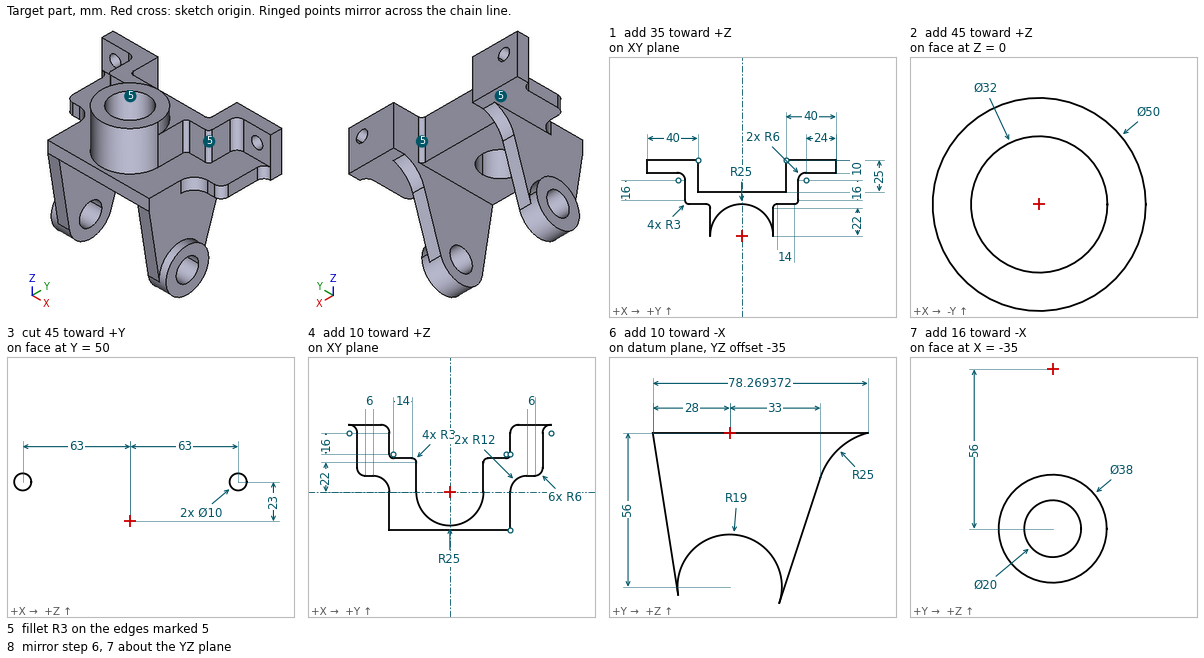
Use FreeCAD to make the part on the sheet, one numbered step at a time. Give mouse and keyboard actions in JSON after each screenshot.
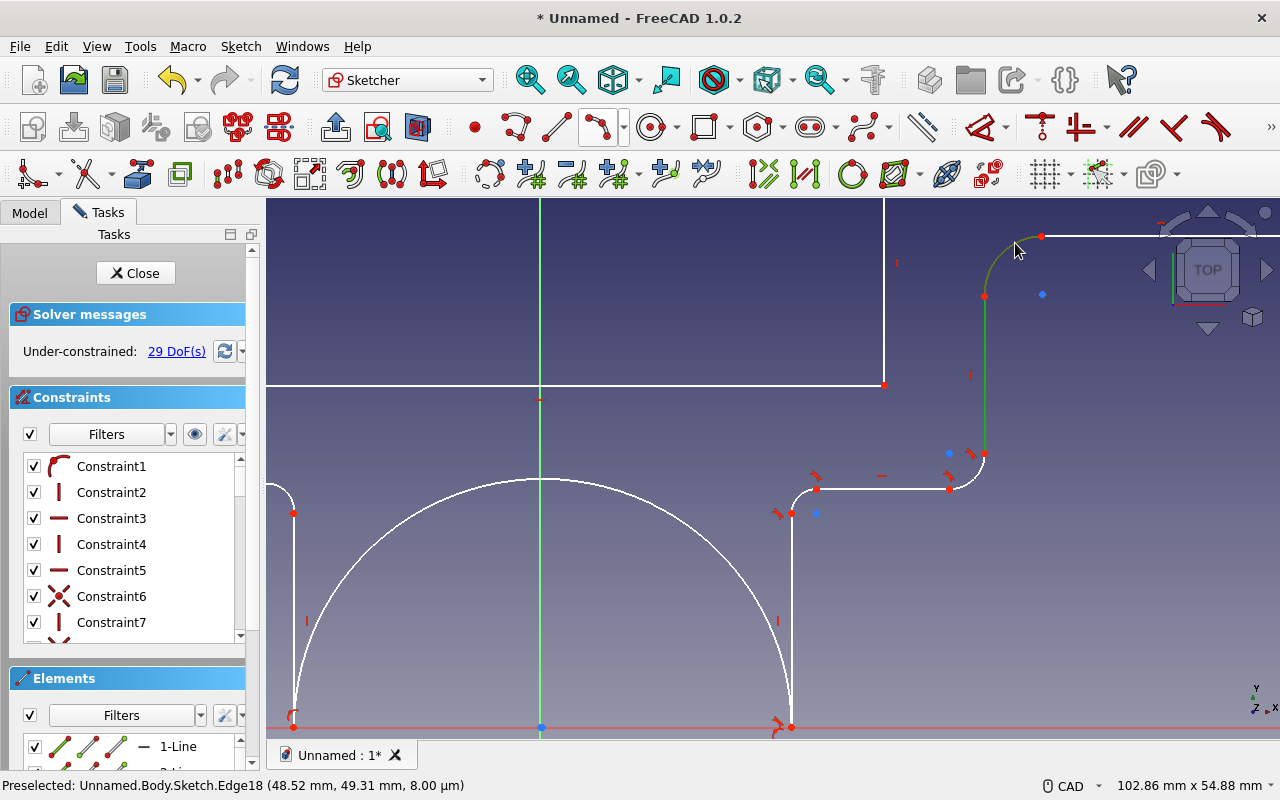
{"action": "left_click", "coordinate": [1216, 128]}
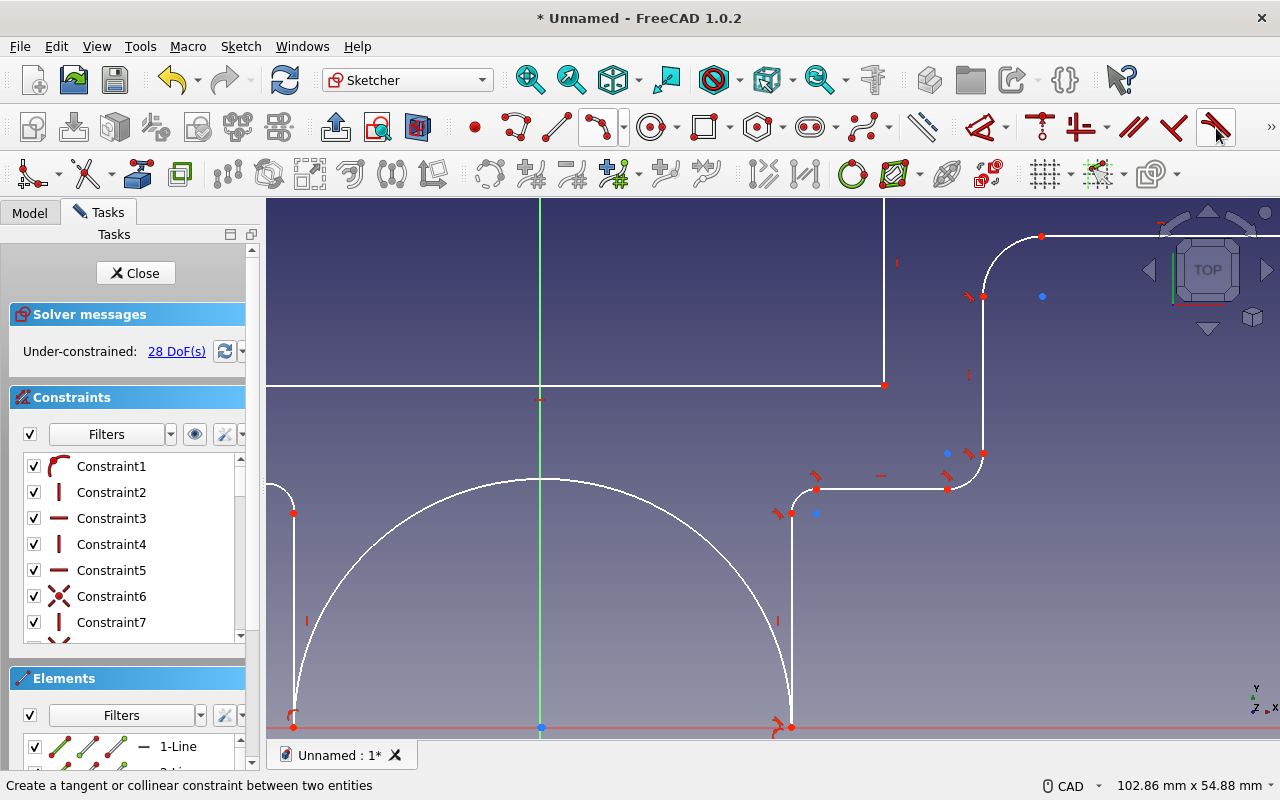
{"action": "left_click", "coordinate": [1114, 236]}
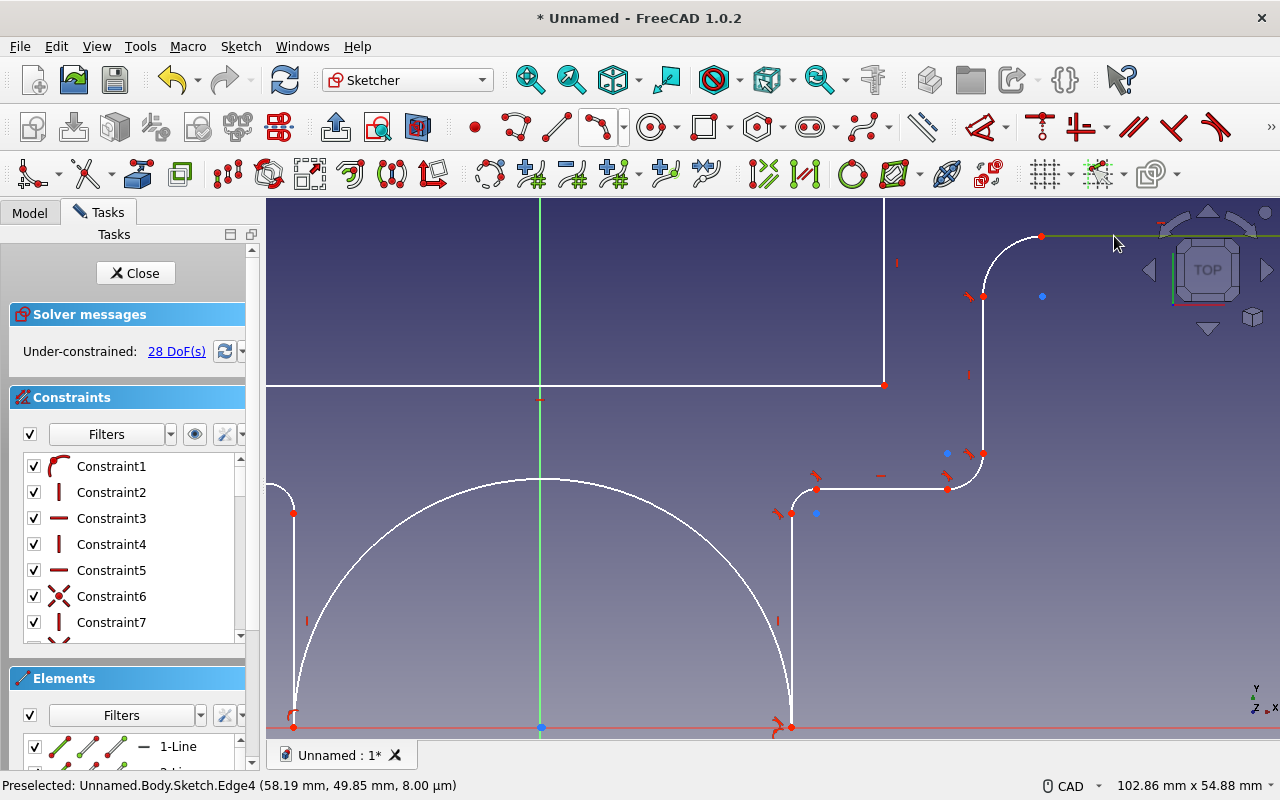
{"action": "left_click", "coordinate": [1015, 243]}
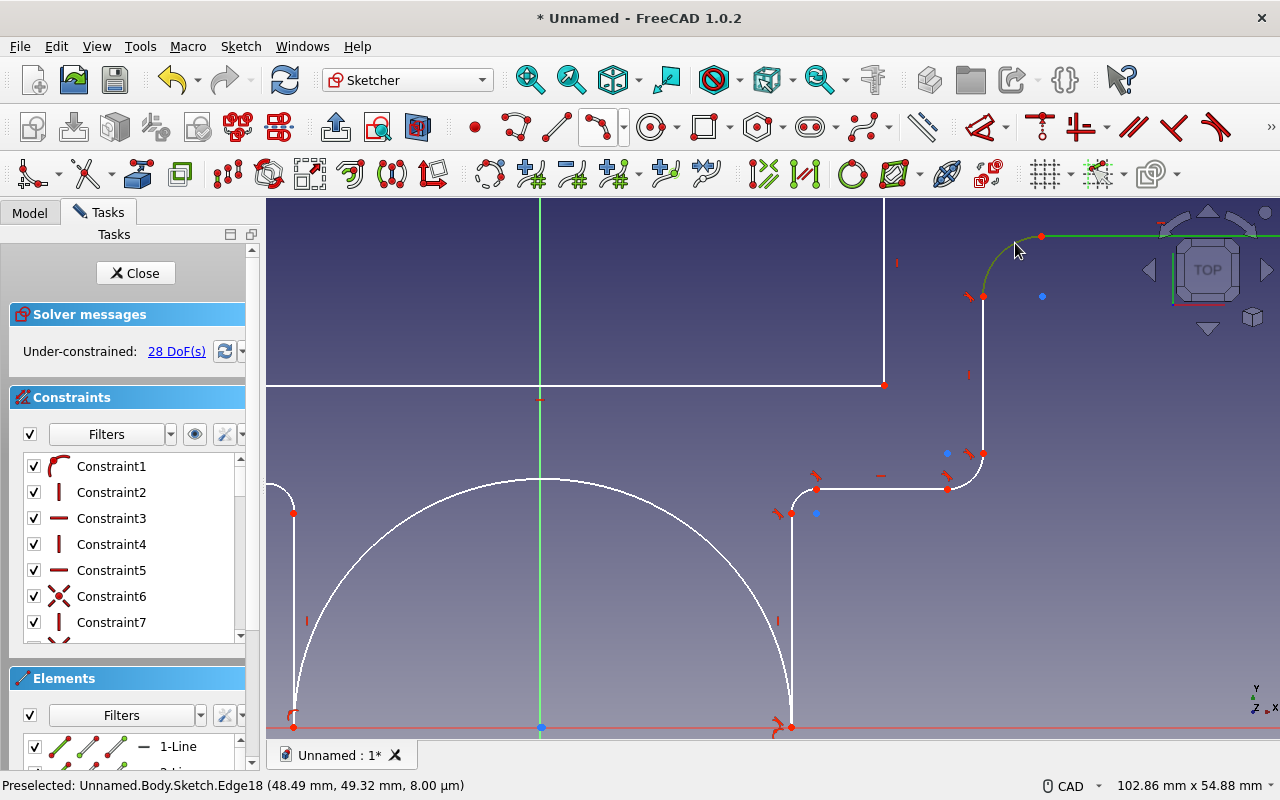
{"action": "left_click", "coordinate": [1216, 128]}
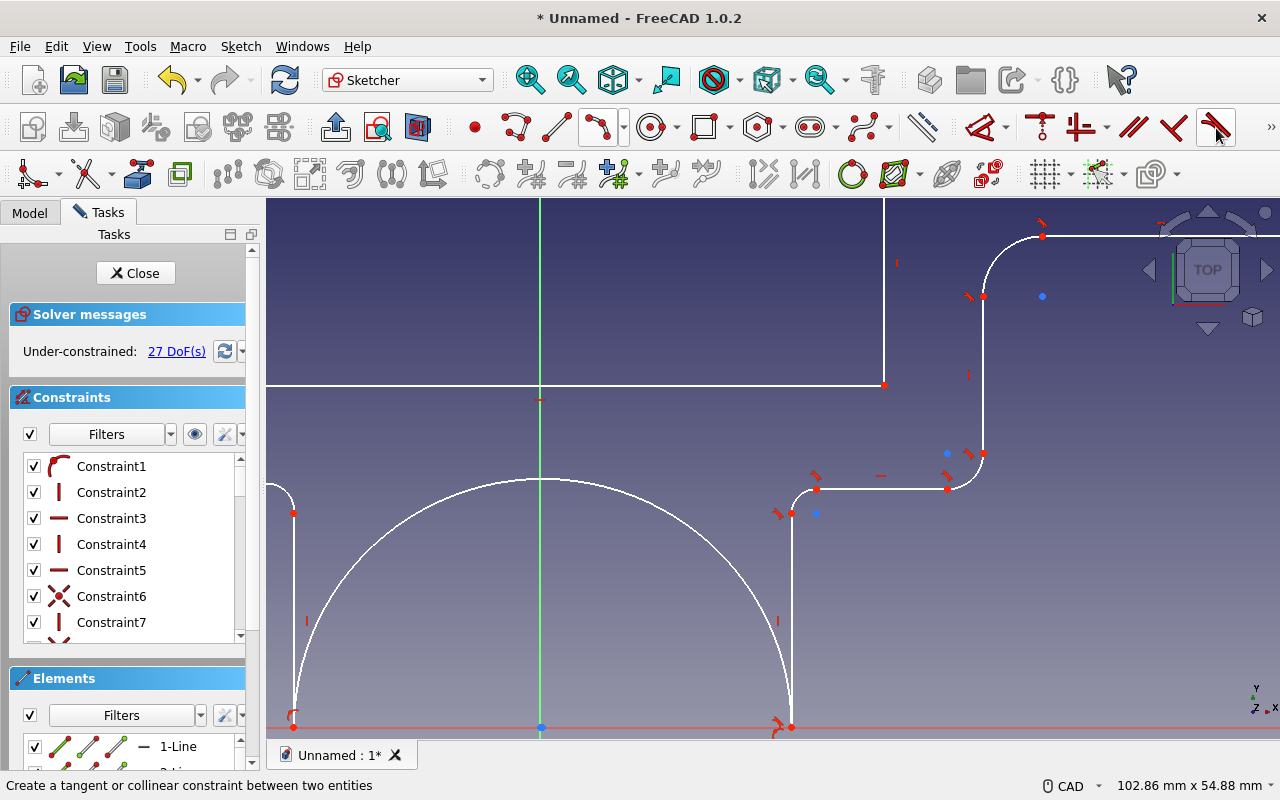
{"action": "scroll", "coordinate": [800, 490], "scroll_direction": "down", "scroll_amount": 5}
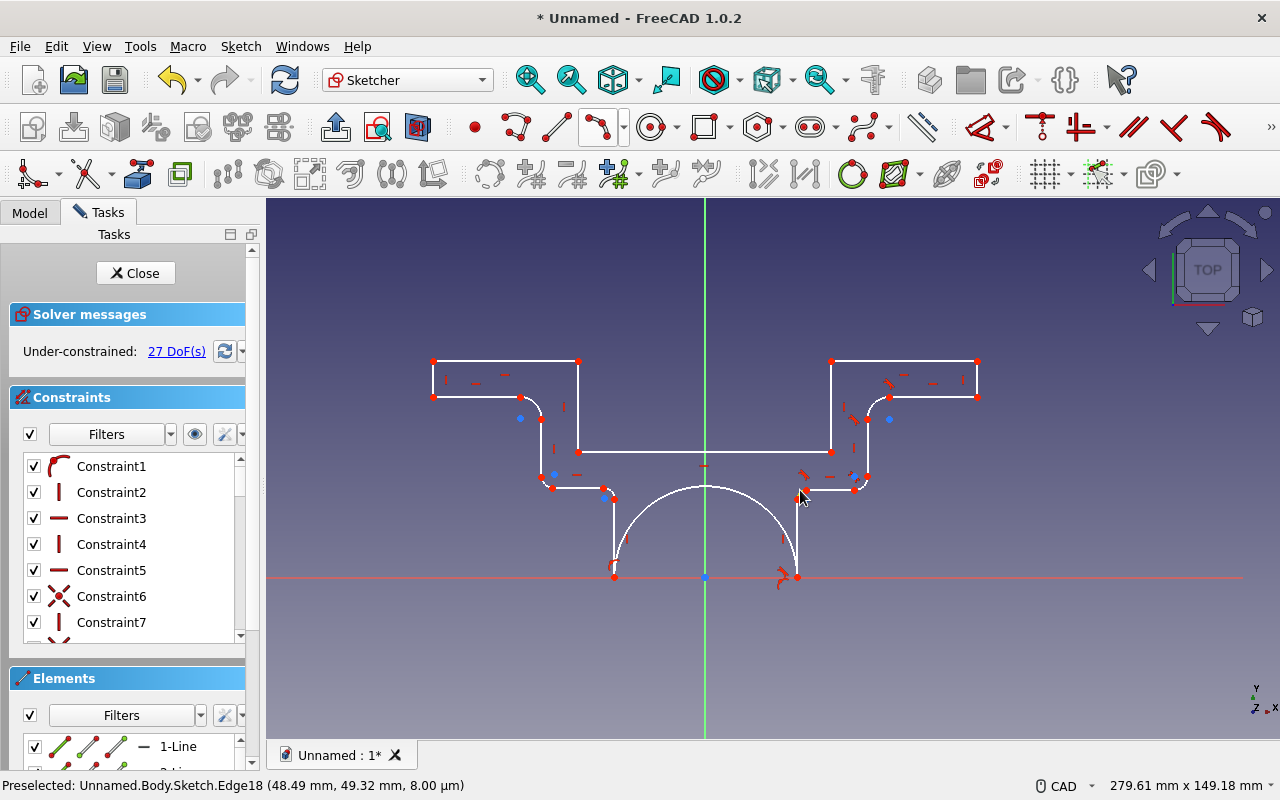
{"action": "left_click", "coordinate": [459, 397]}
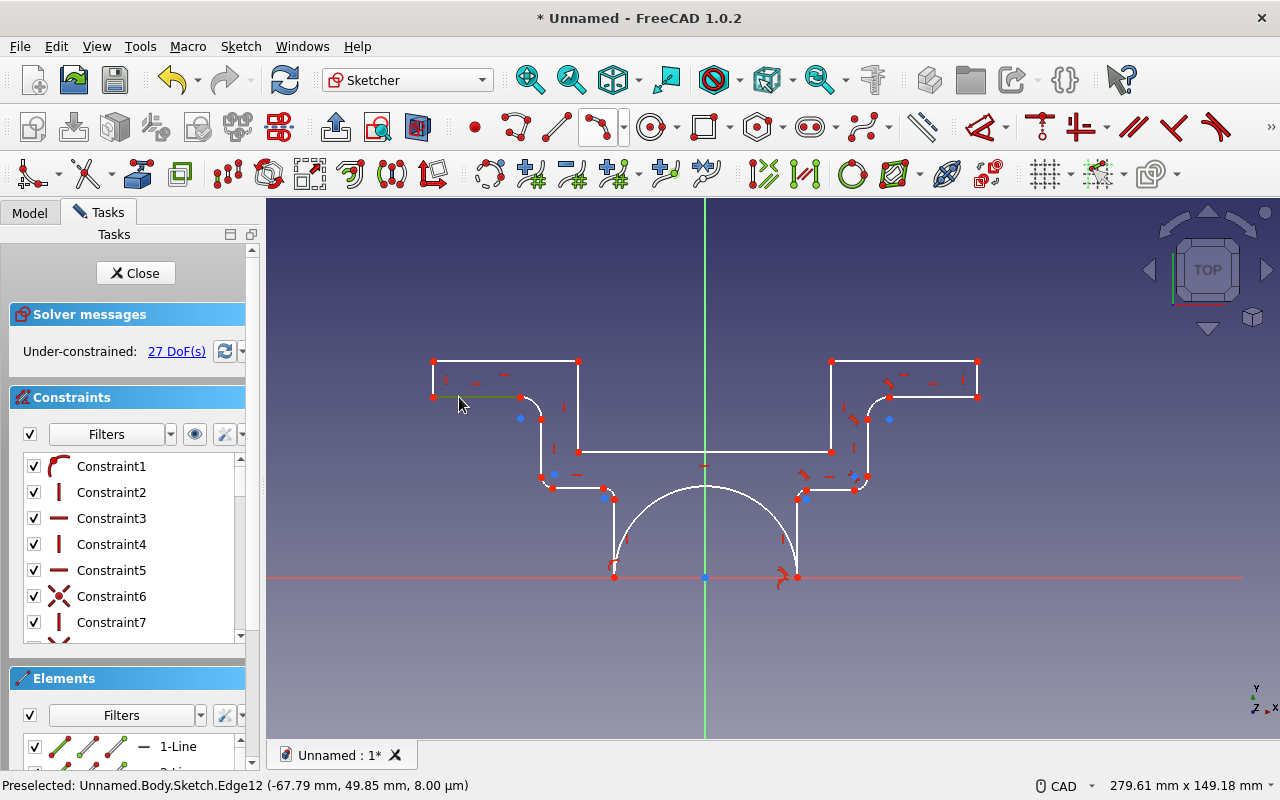
{"action": "scroll", "coordinate": [539, 409], "scroll_direction": "up", "scroll_amount": 2}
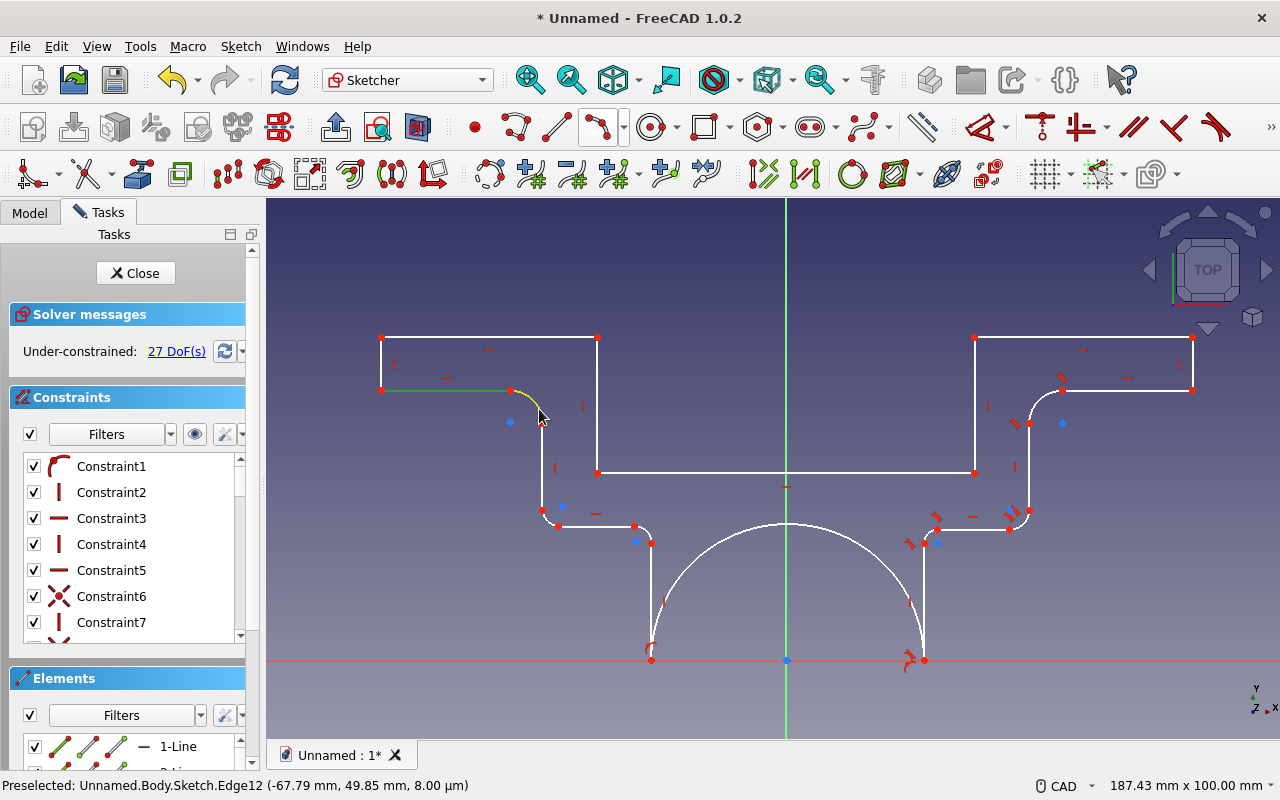
{"action": "left_click", "coordinate": [539, 409]}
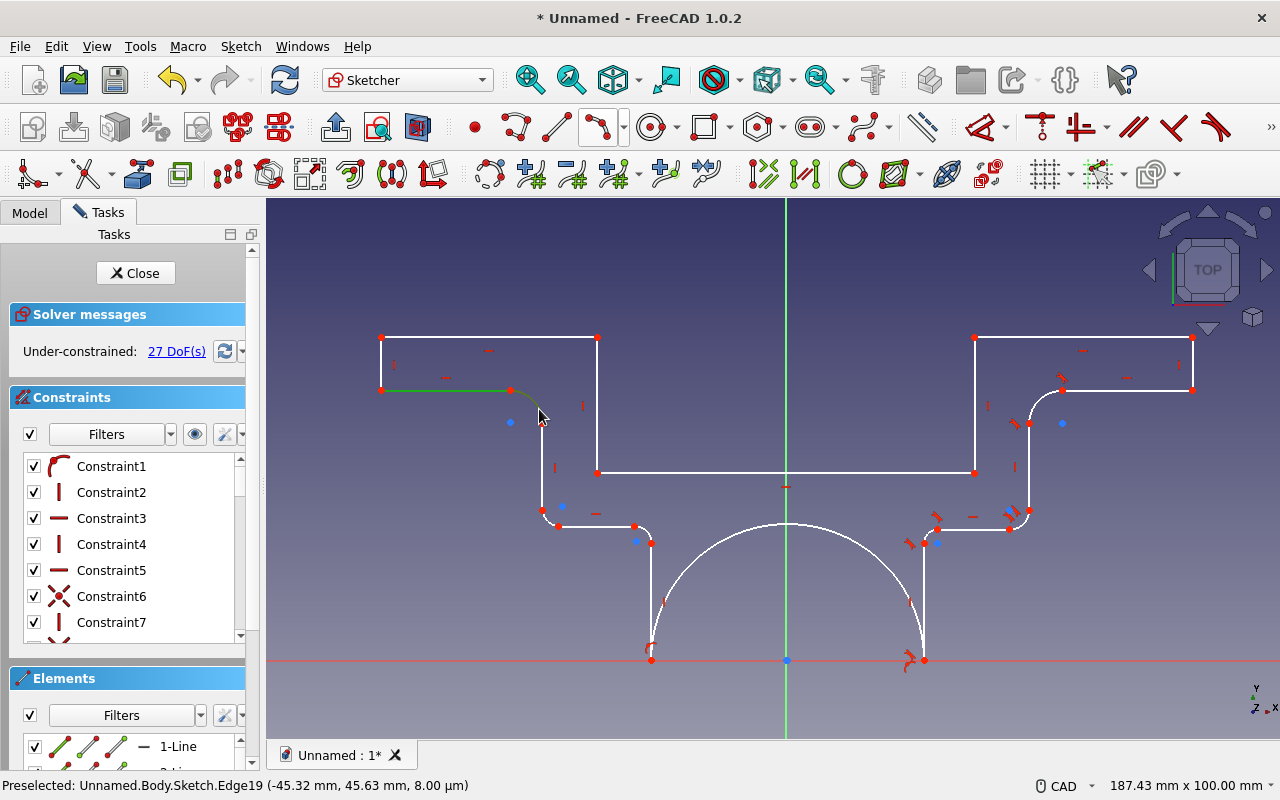
{"action": "left_click", "coordinate": [1216, 128]}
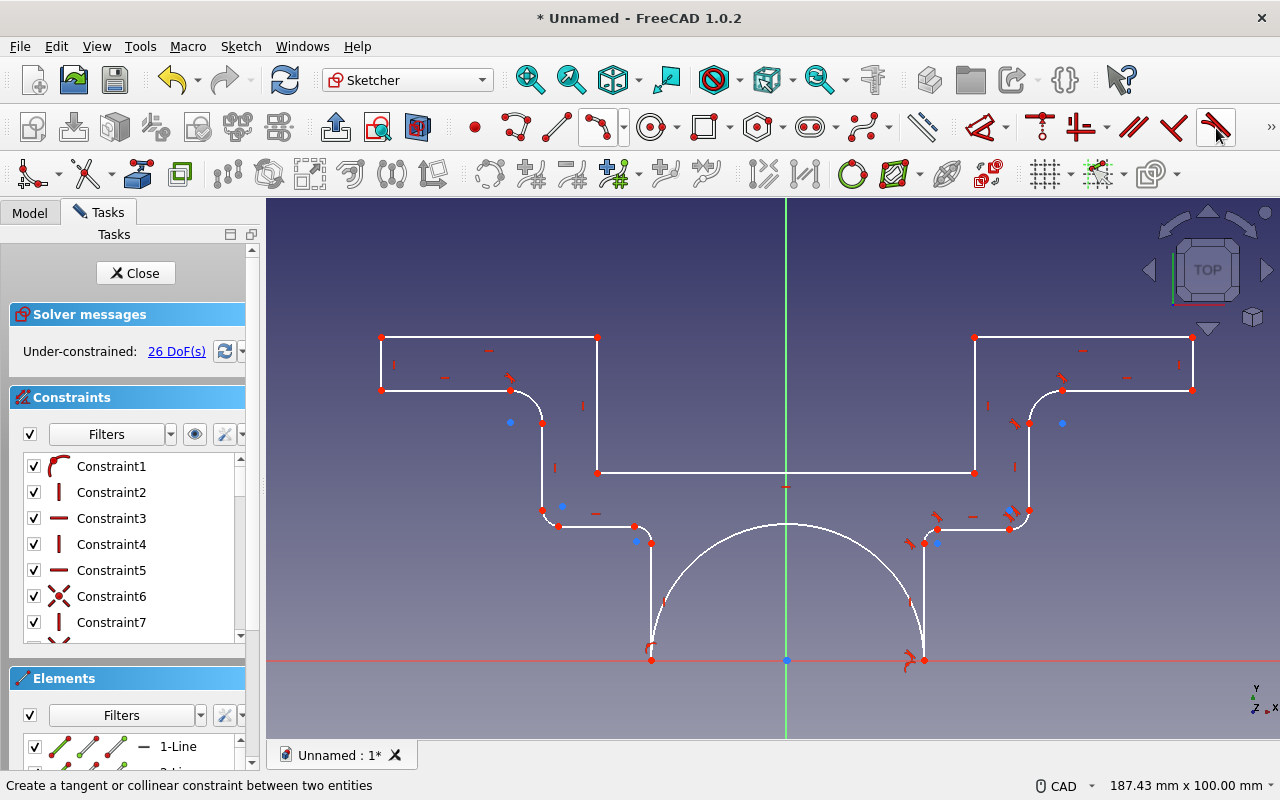
{"action": "left_click", "coordinate": [542, 450]}